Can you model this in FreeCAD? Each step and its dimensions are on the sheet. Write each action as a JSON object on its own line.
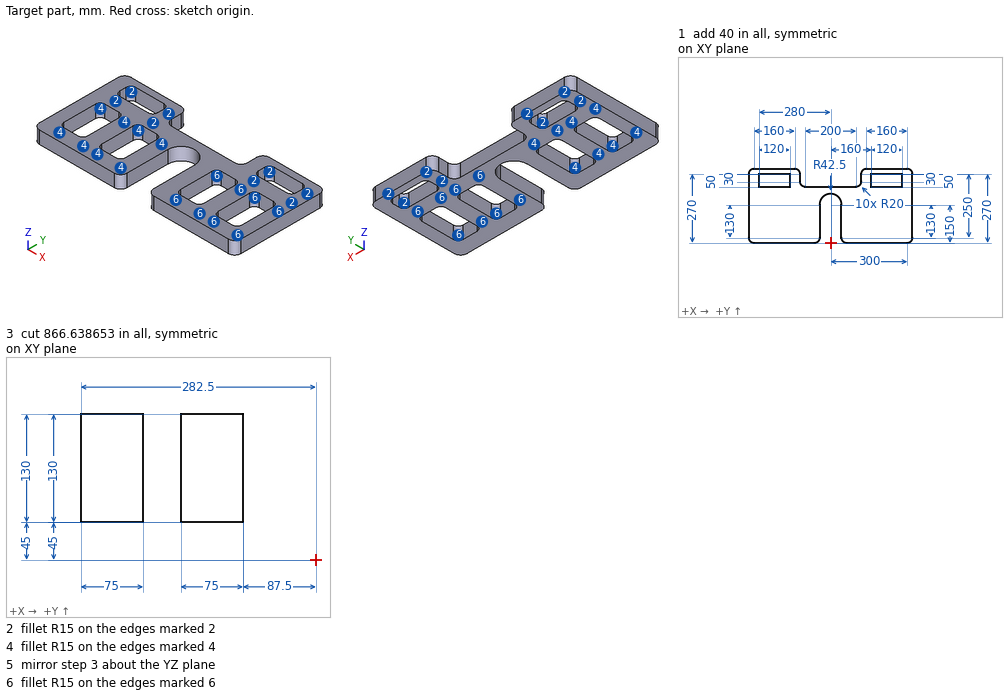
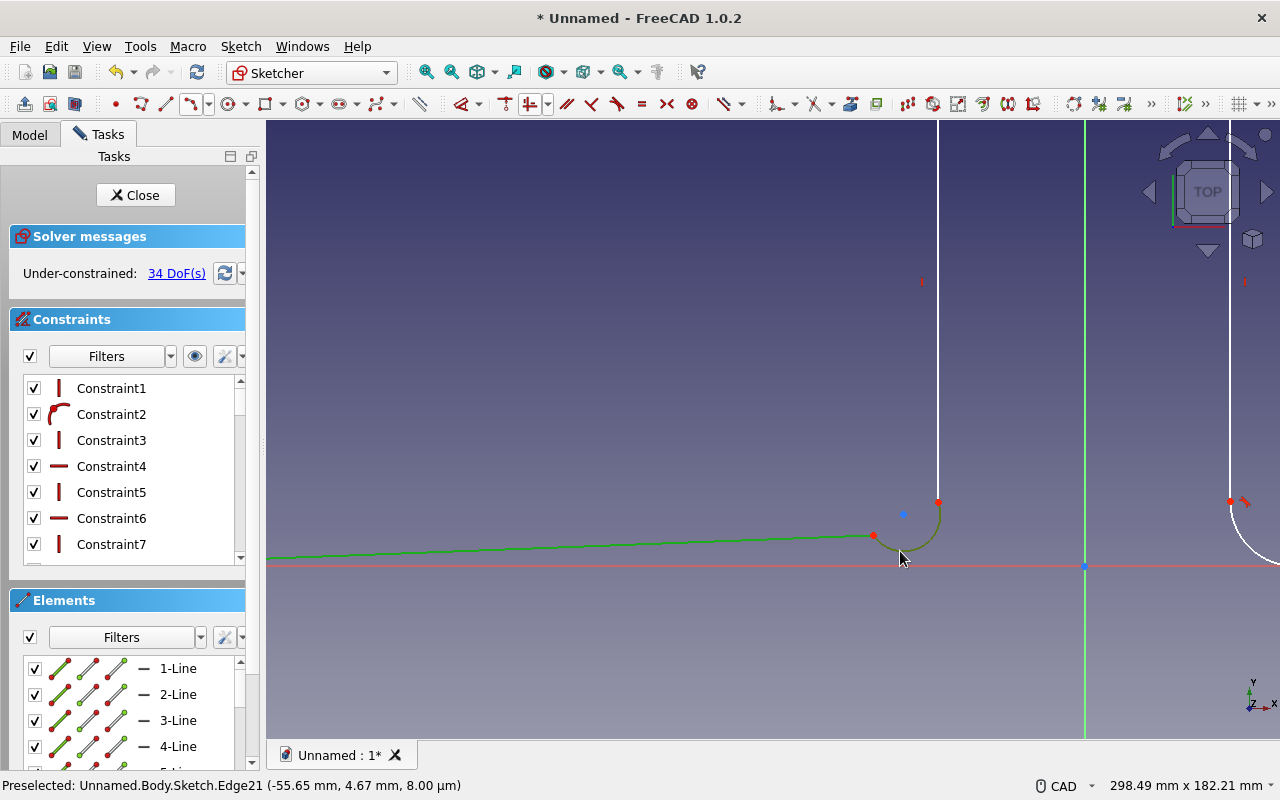
{"action": "key", "text": "t"}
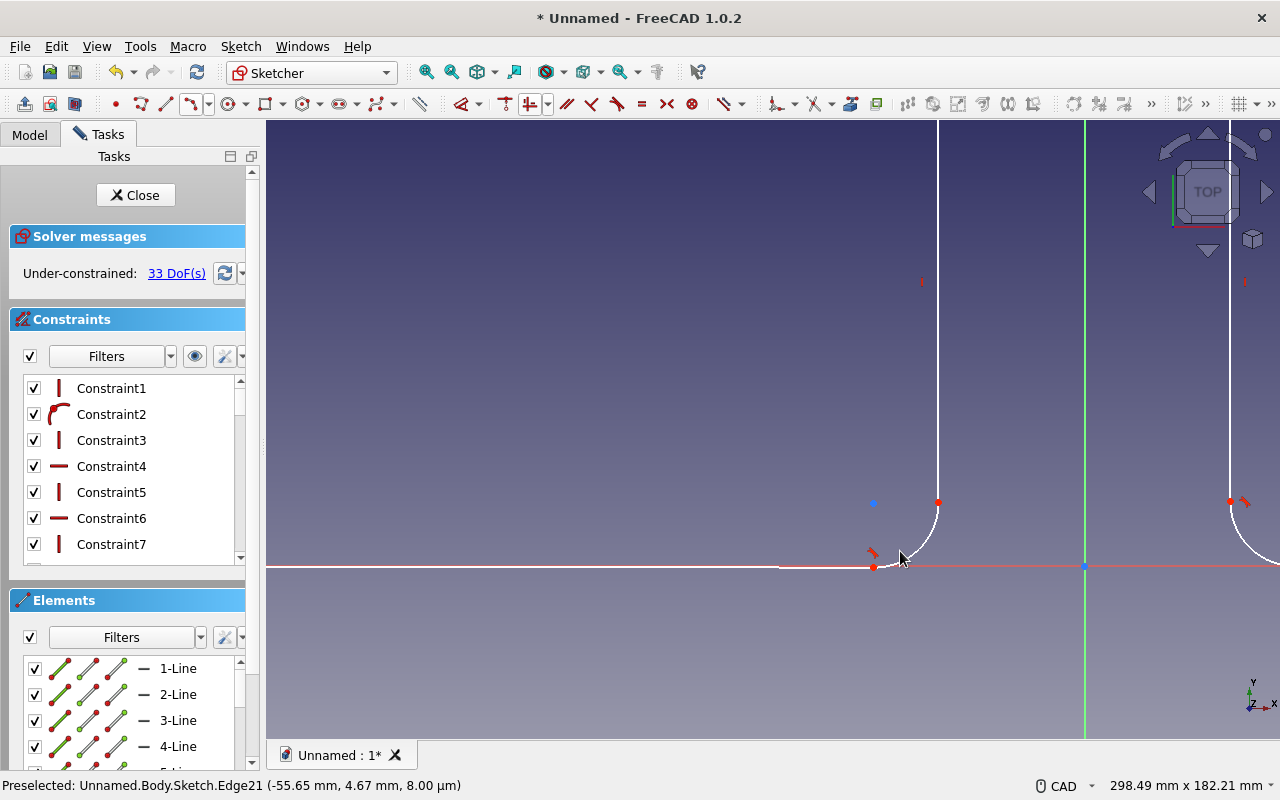
{"action": "scroll", "coordinate": [580, 546], "scroll_direction": "down", "scroll_amount": 7}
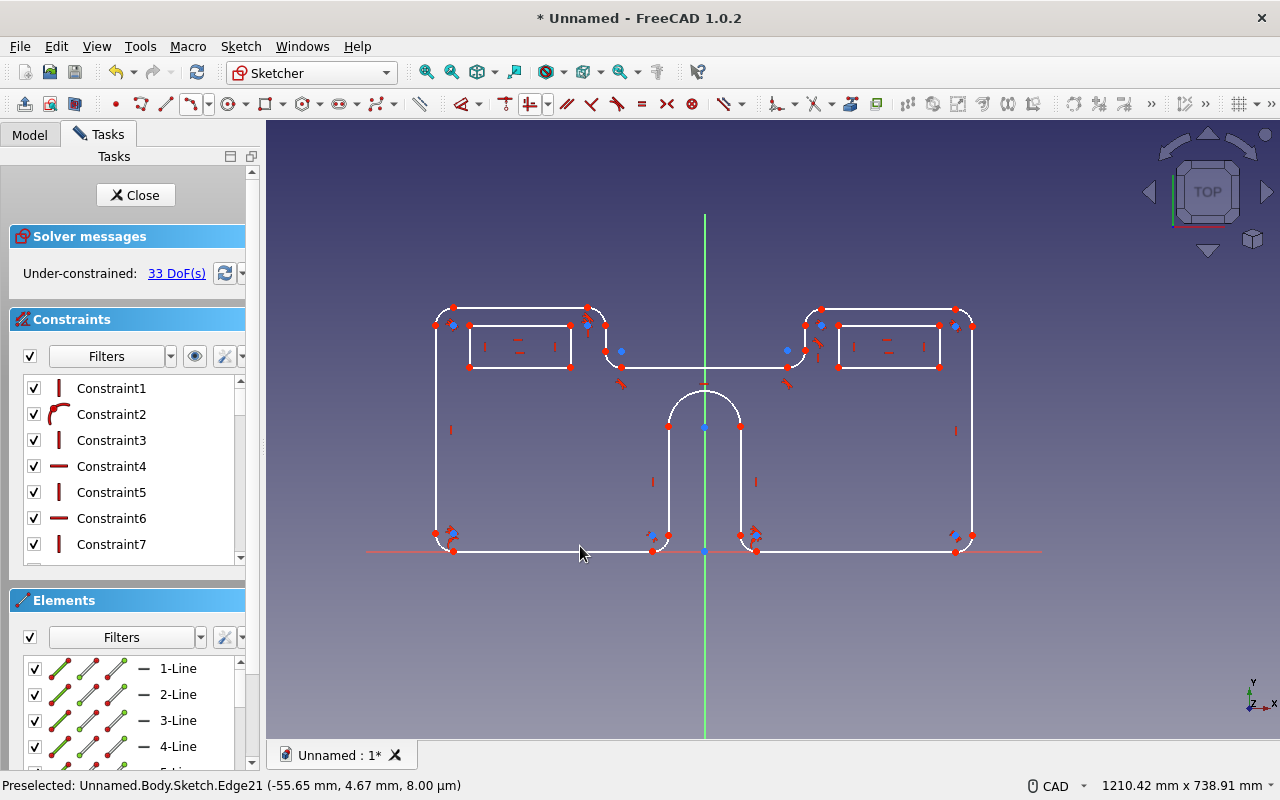
{"action": "left_click", "coordinate": [669, 503]}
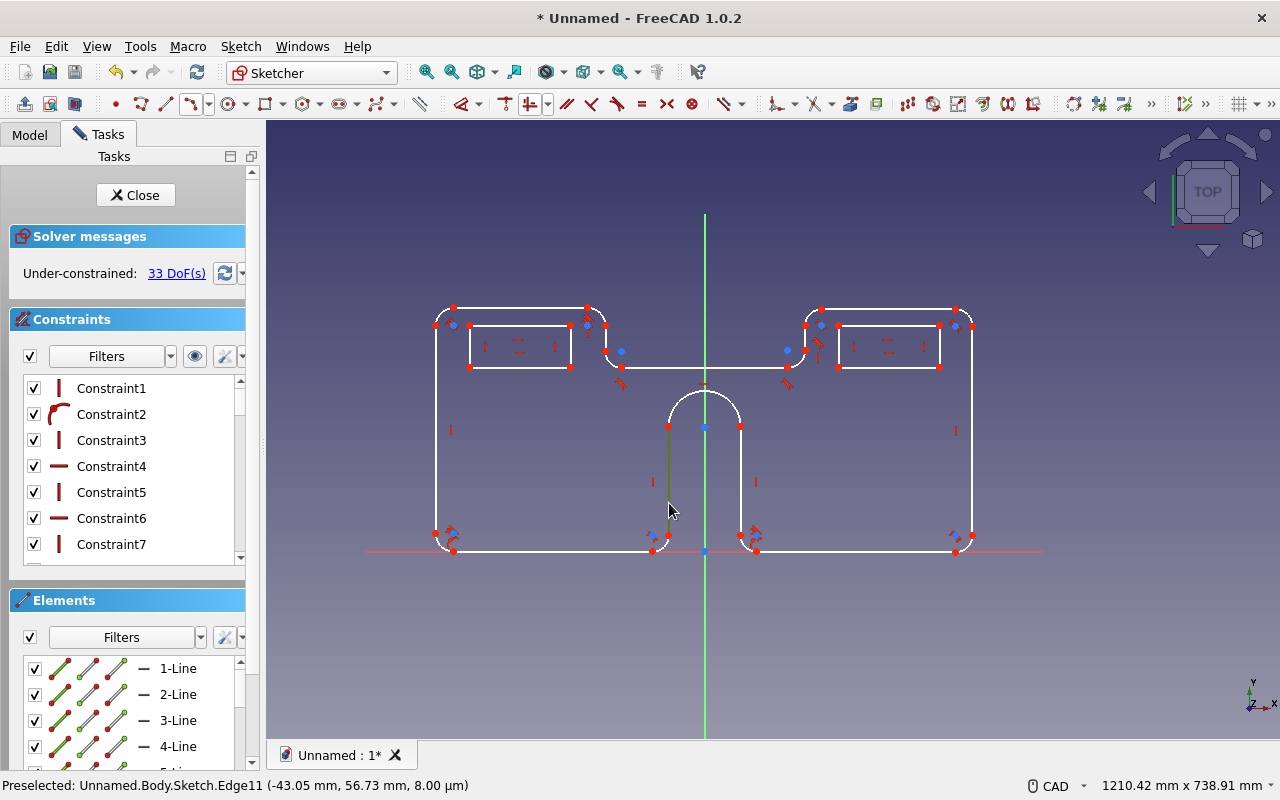
{"action": "scroll", "coordinate": [660, 550], "scroll_direction": "up", "scroll_amount": 4}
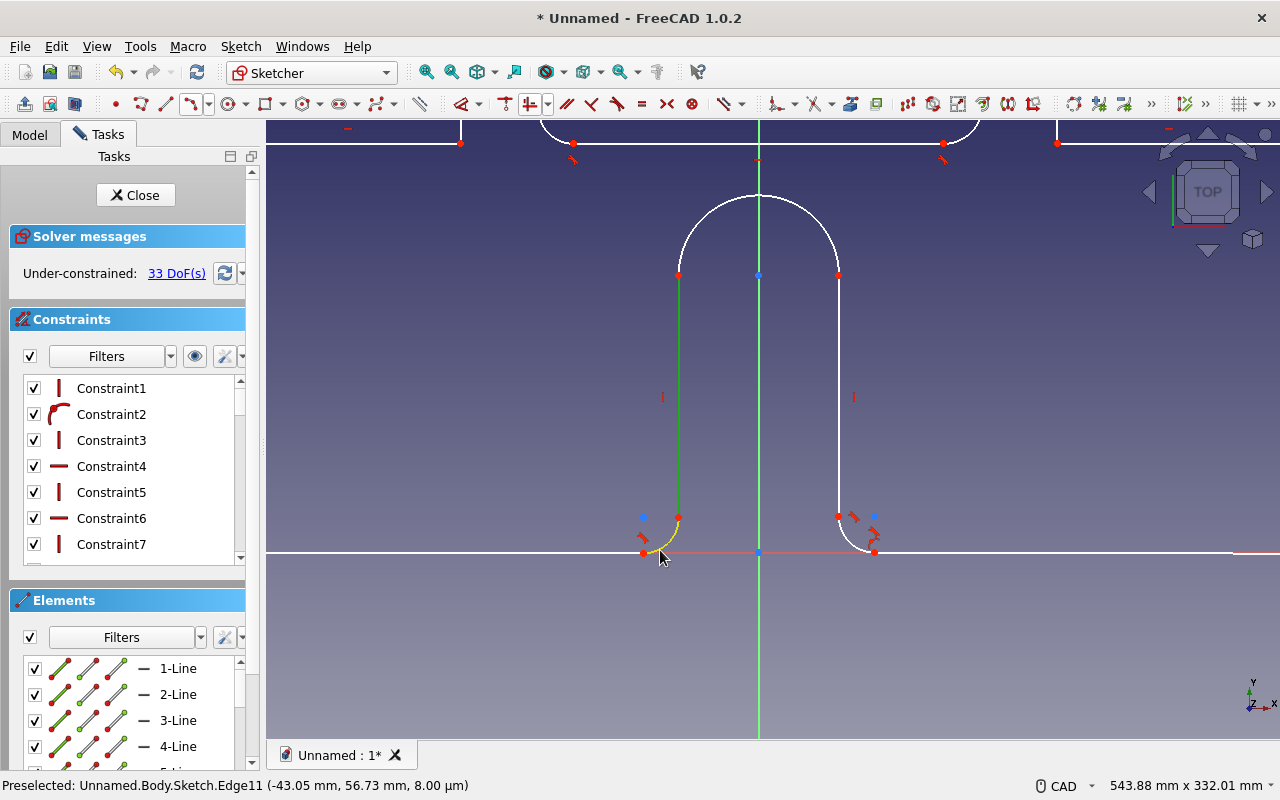
{"action": "left_click", "coordinate": [659, 549]}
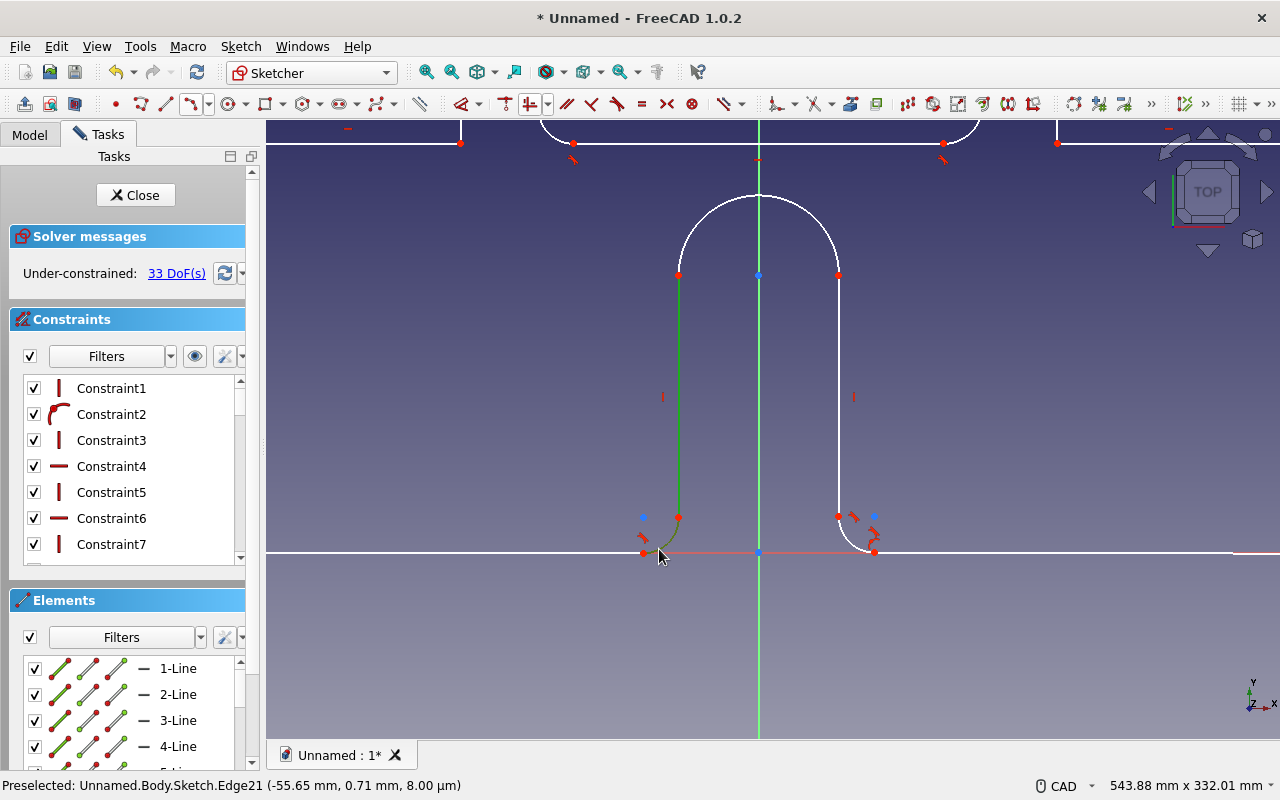
{"action": "key", "text": "t"}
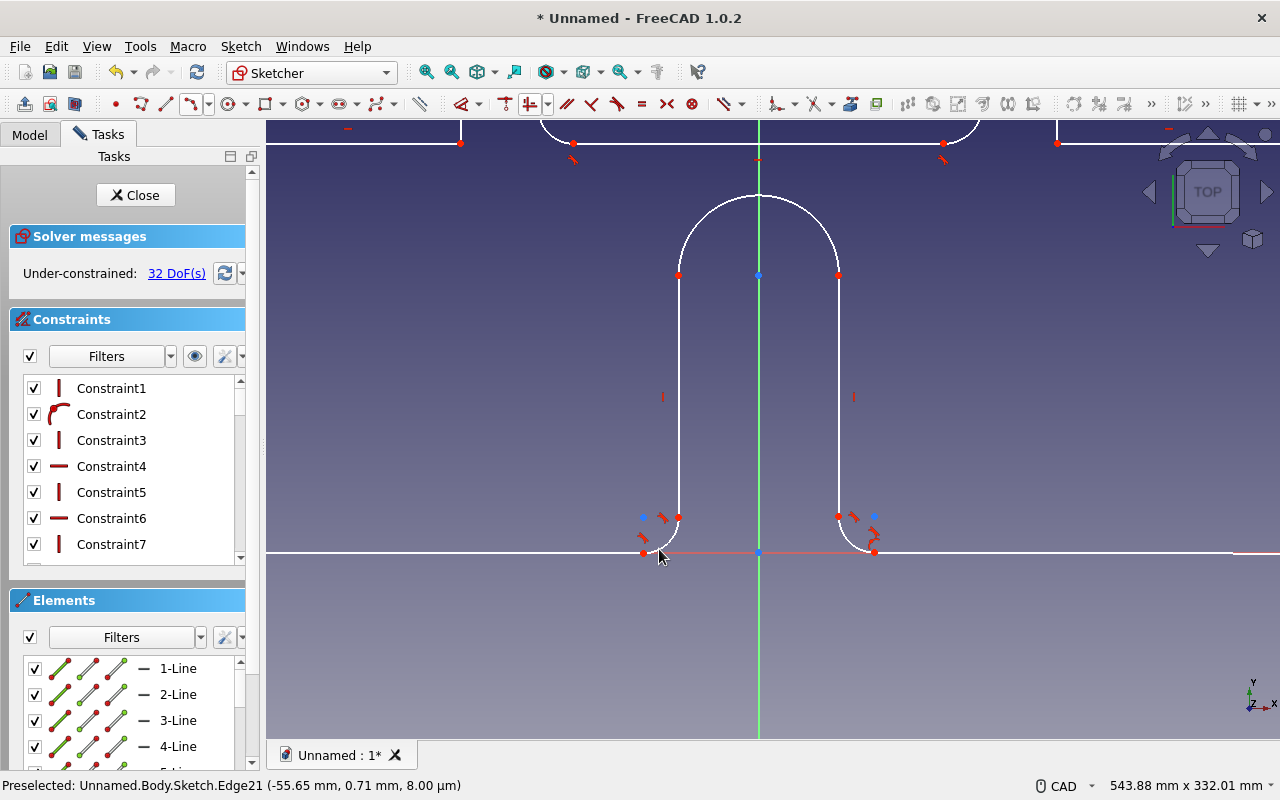
{"action": "left_click", "coordinate": [1007, 553]}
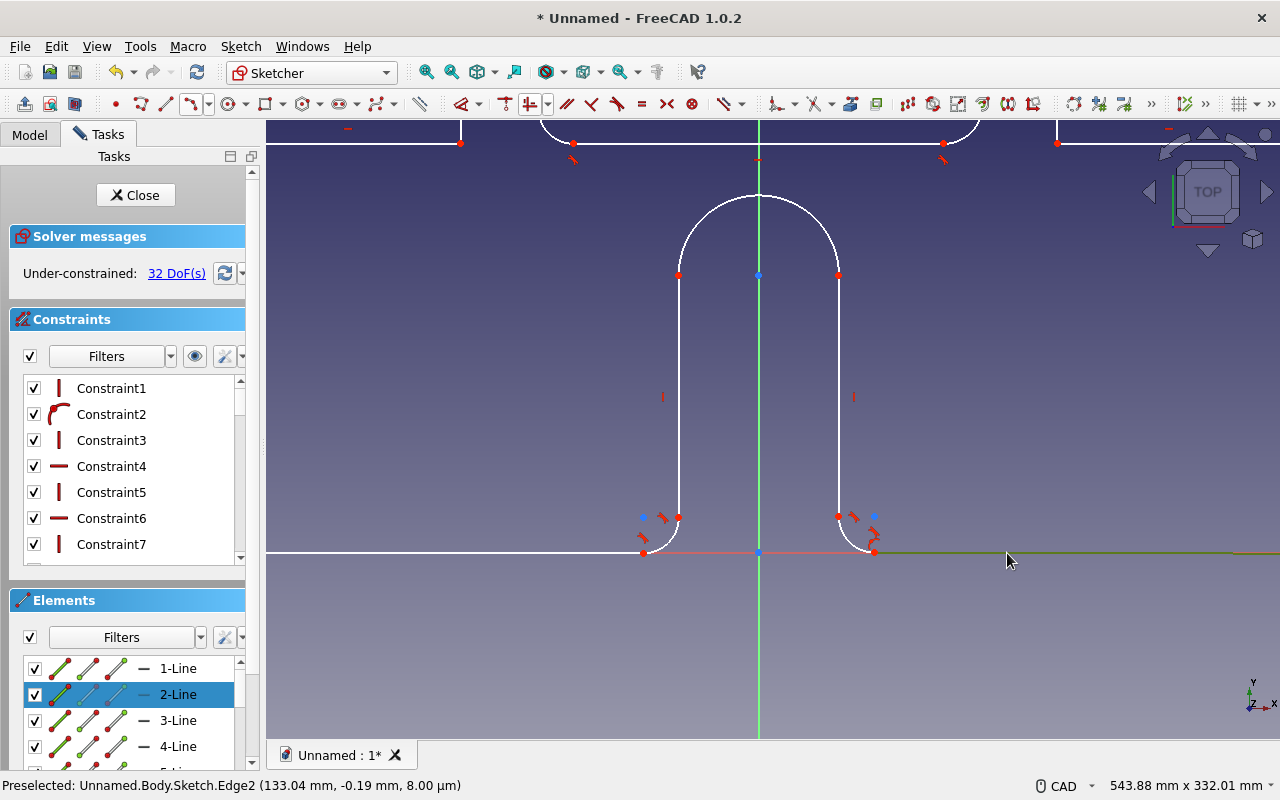
{"action": "key", "text": "h"}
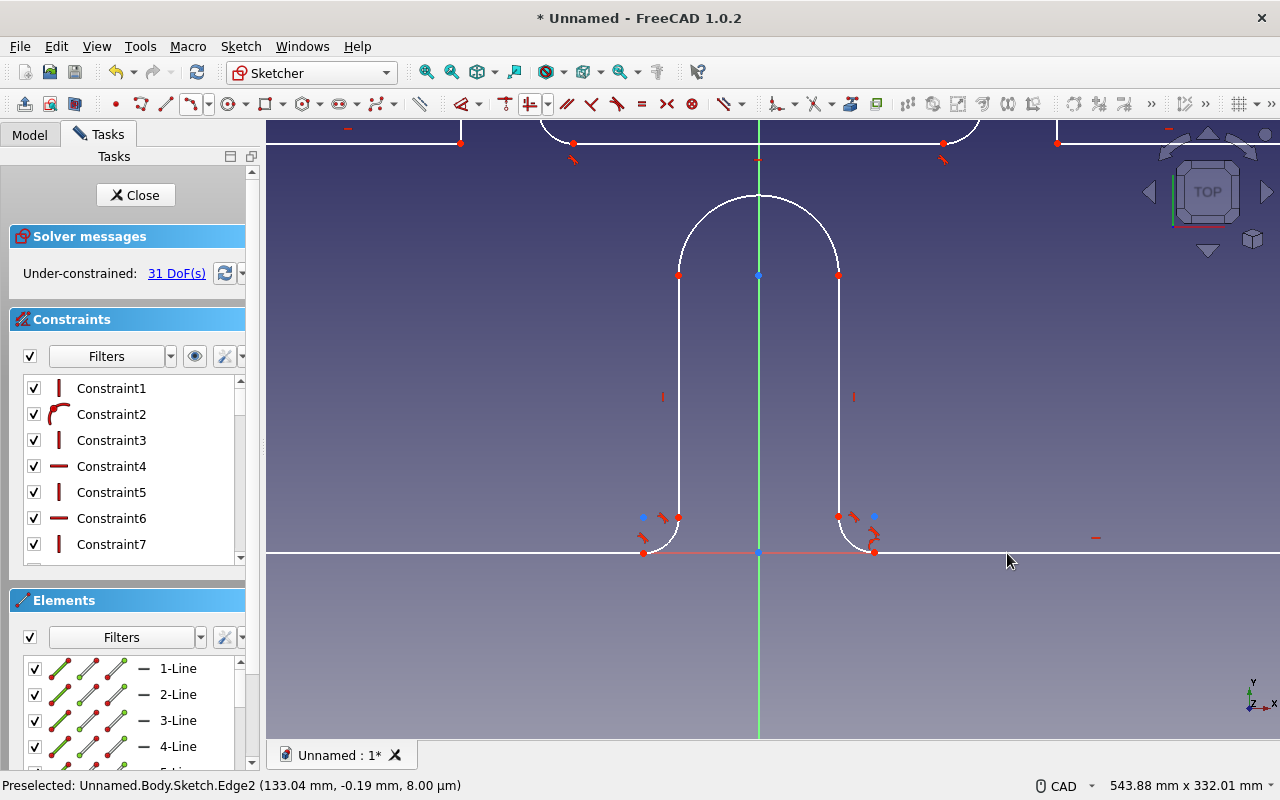
{"action": "left_click", "coordinate": [333, 553]}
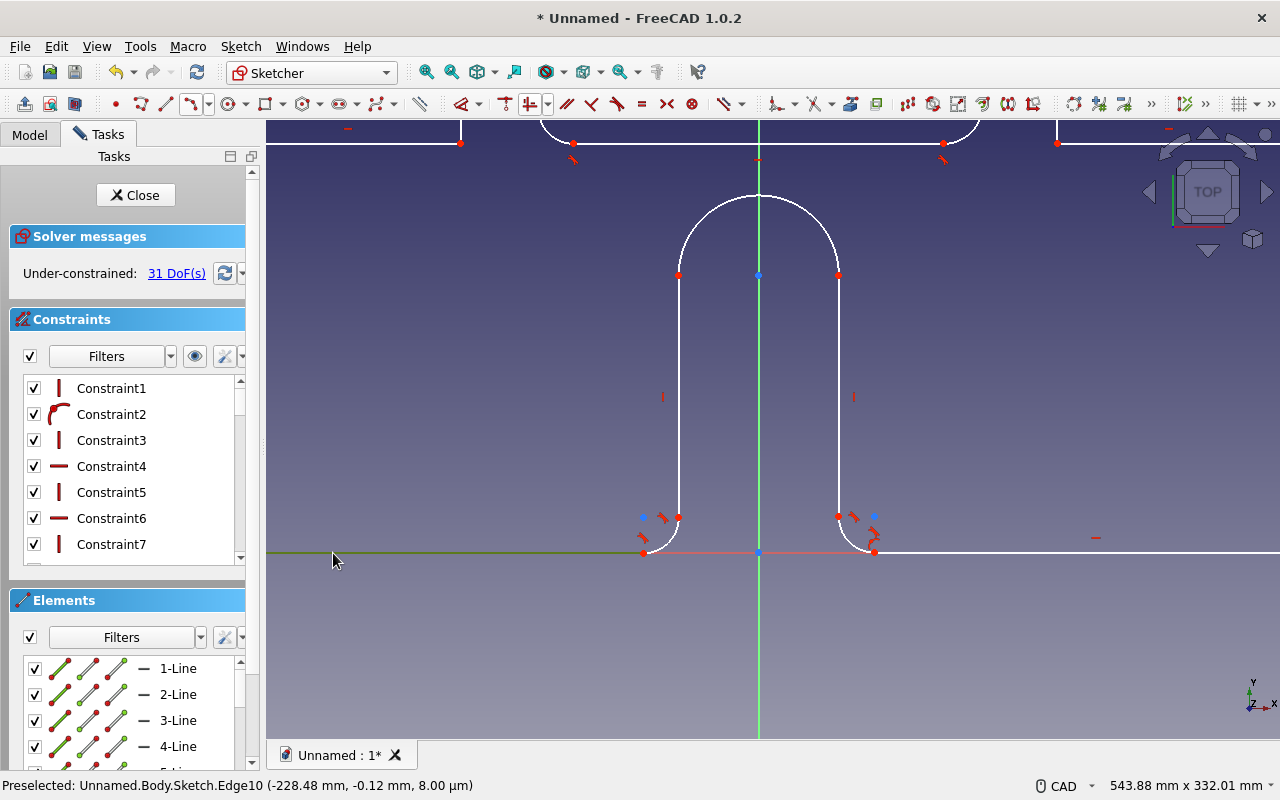
{"action": "key", "text": "h"}